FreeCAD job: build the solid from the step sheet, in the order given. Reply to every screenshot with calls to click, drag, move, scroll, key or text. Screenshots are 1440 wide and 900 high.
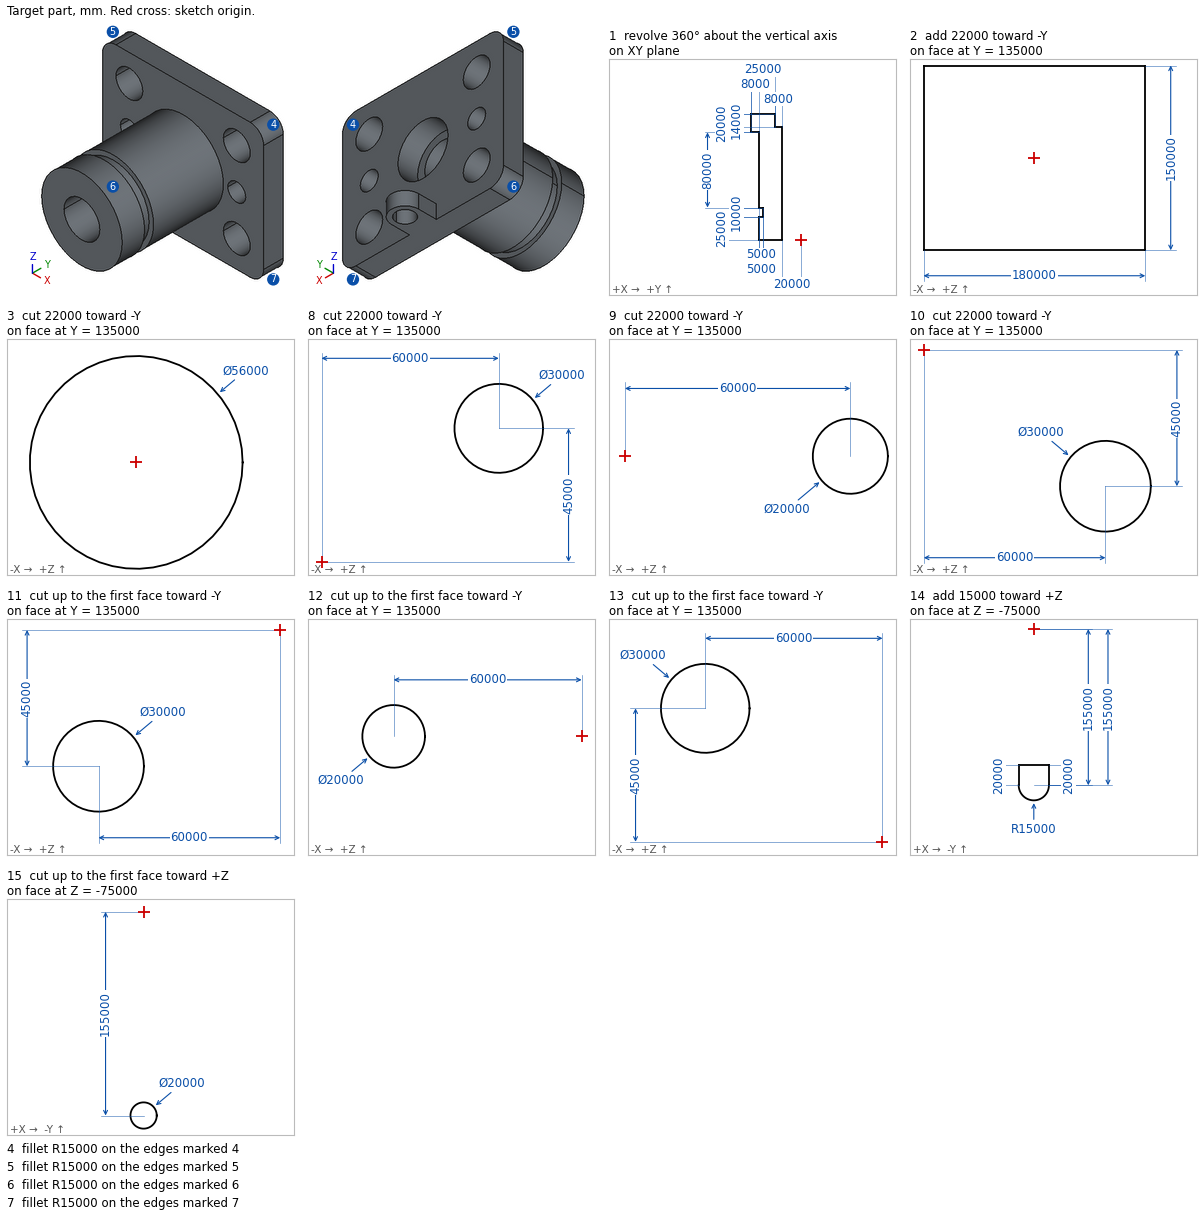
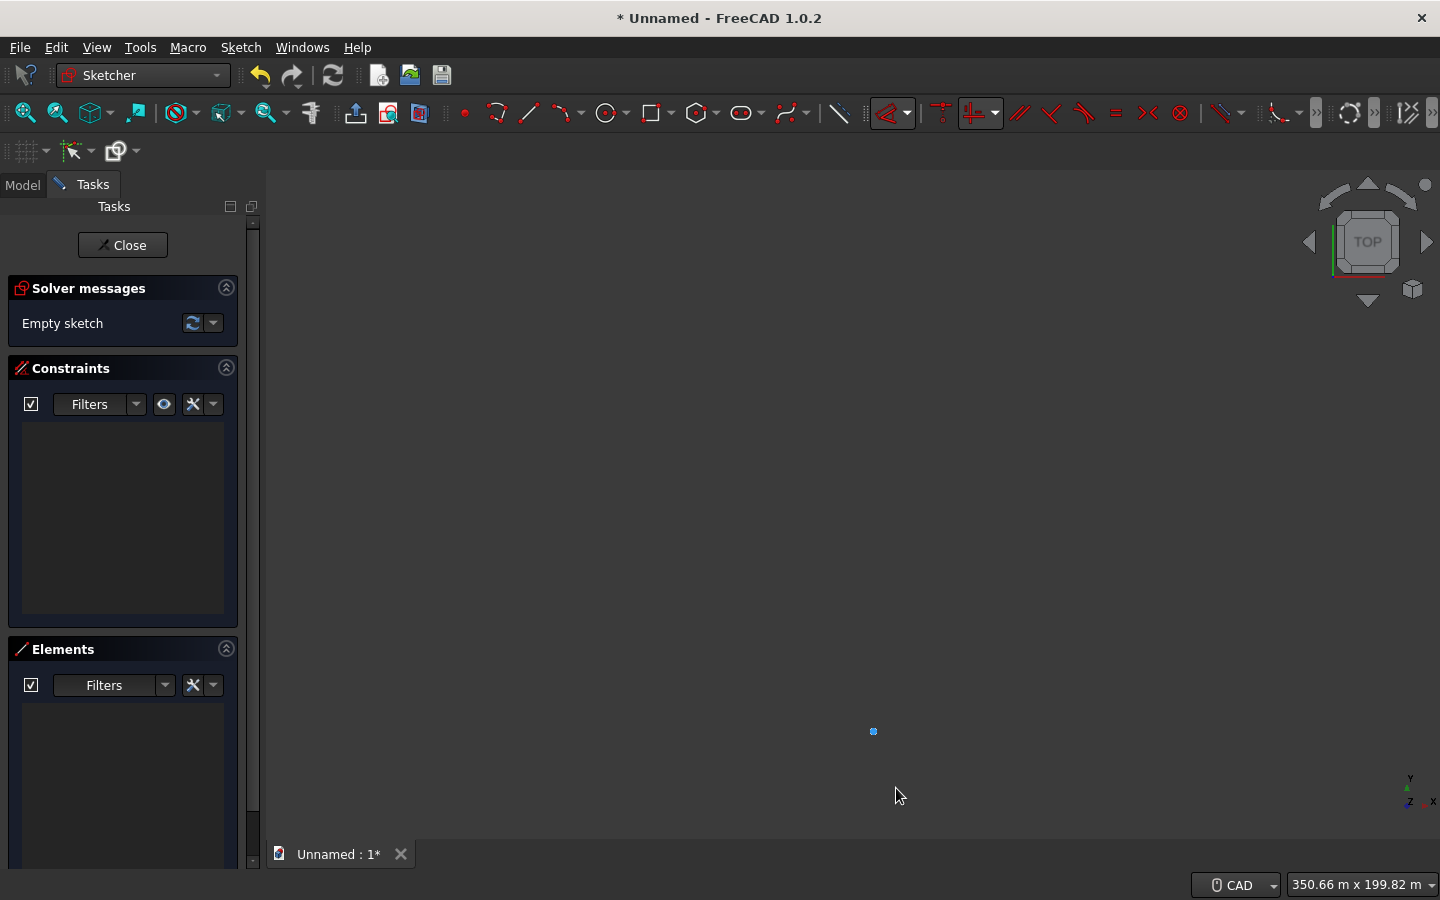
click(498, 114)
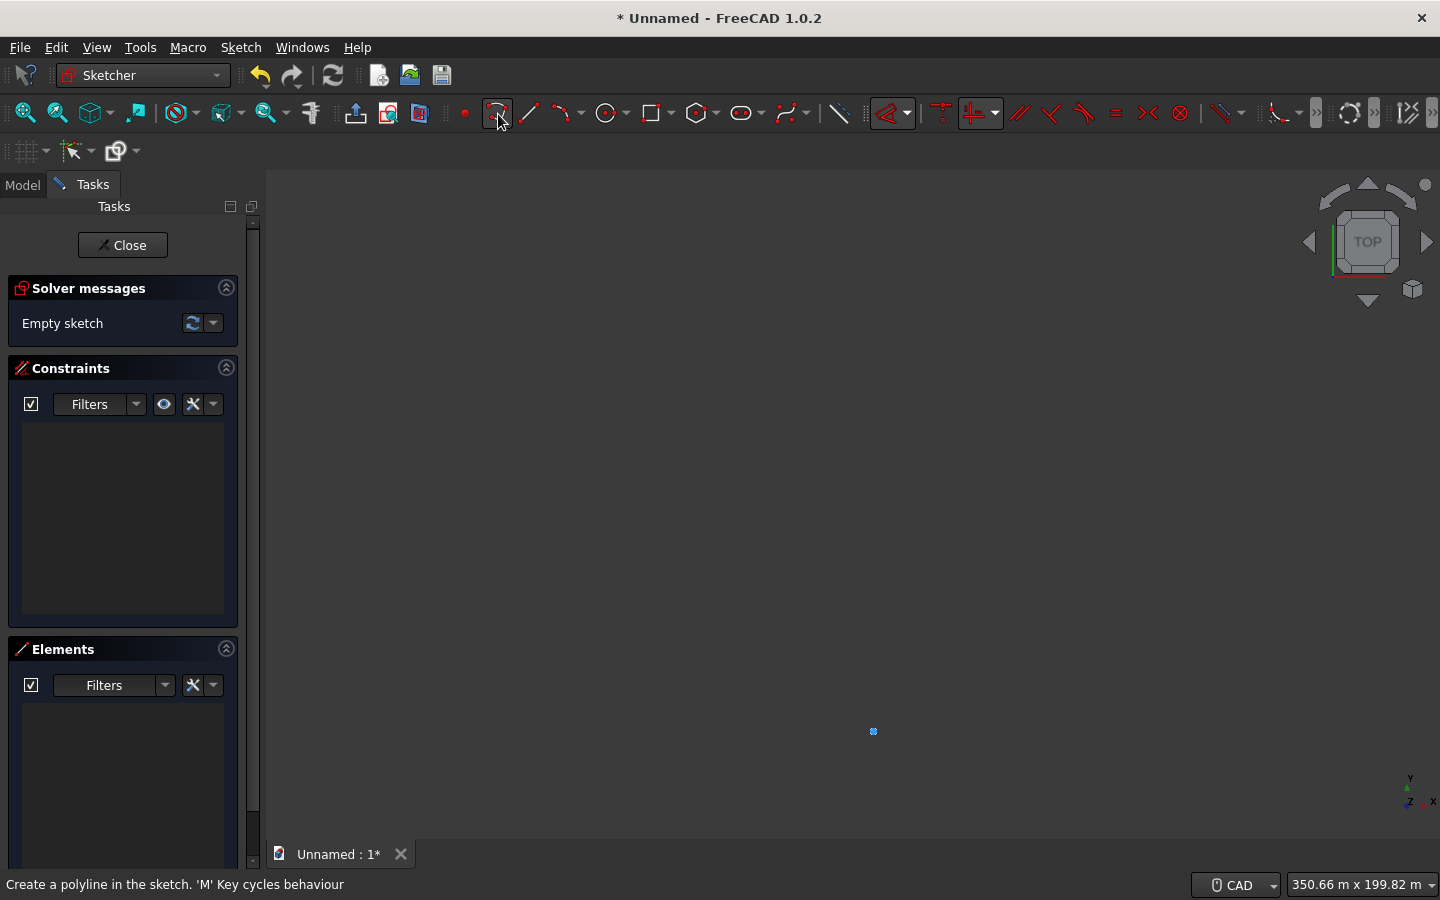
click(807, 732)
click(807, 326)
click(780, 326)
click(780, 280)
click(696, 280)
click(696, 346)
click(723, 346)
click(723, 614)
click(740, 614)
click(740, 648)
click(723, 648)
click(723, 723)
click(807, 733)
key(Escape)
key(Escape)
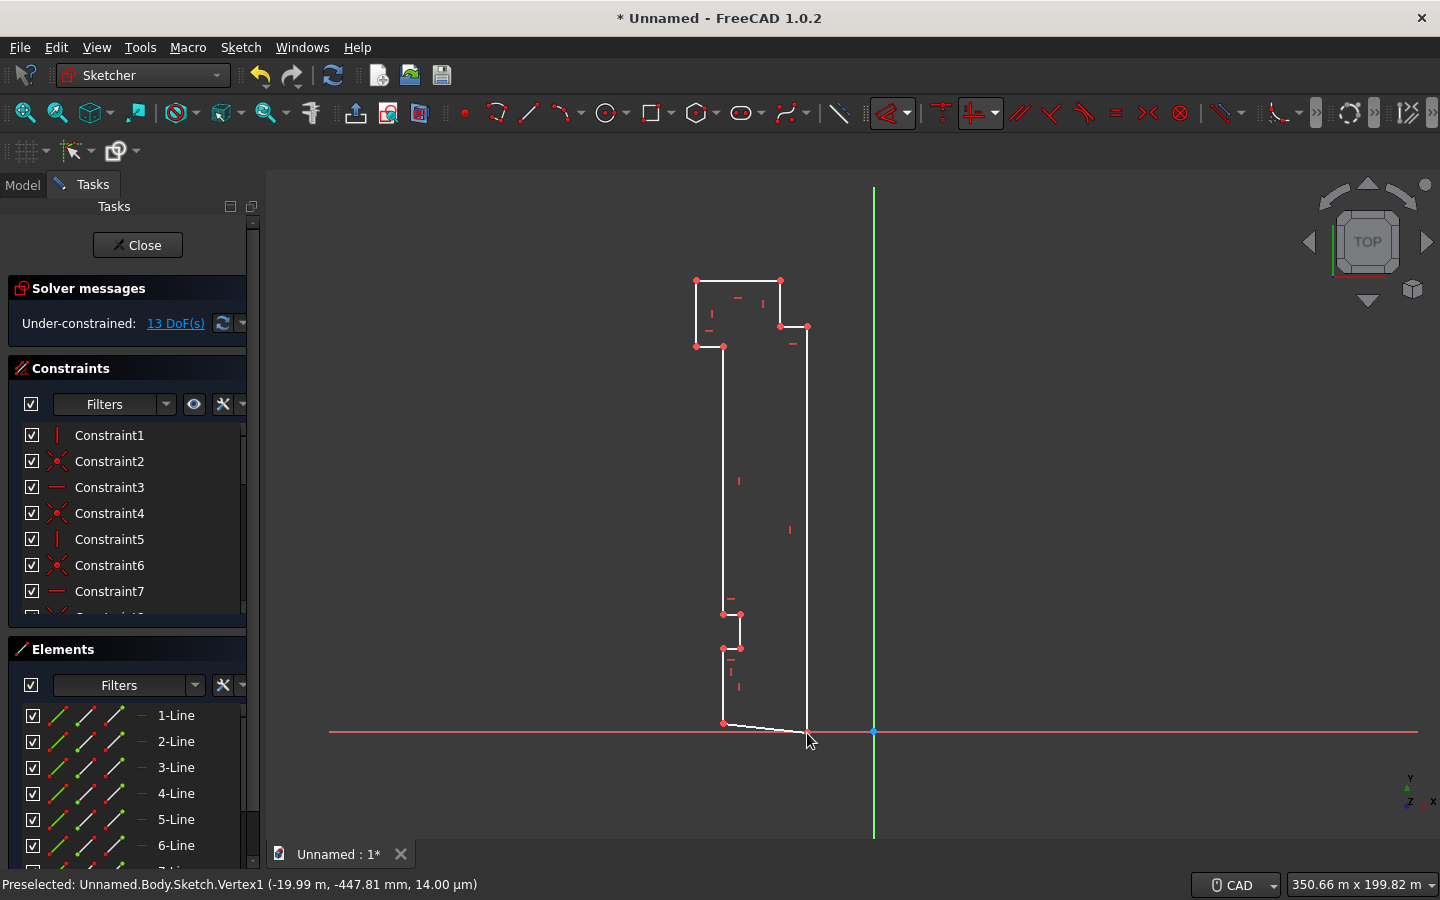
click(782, 730)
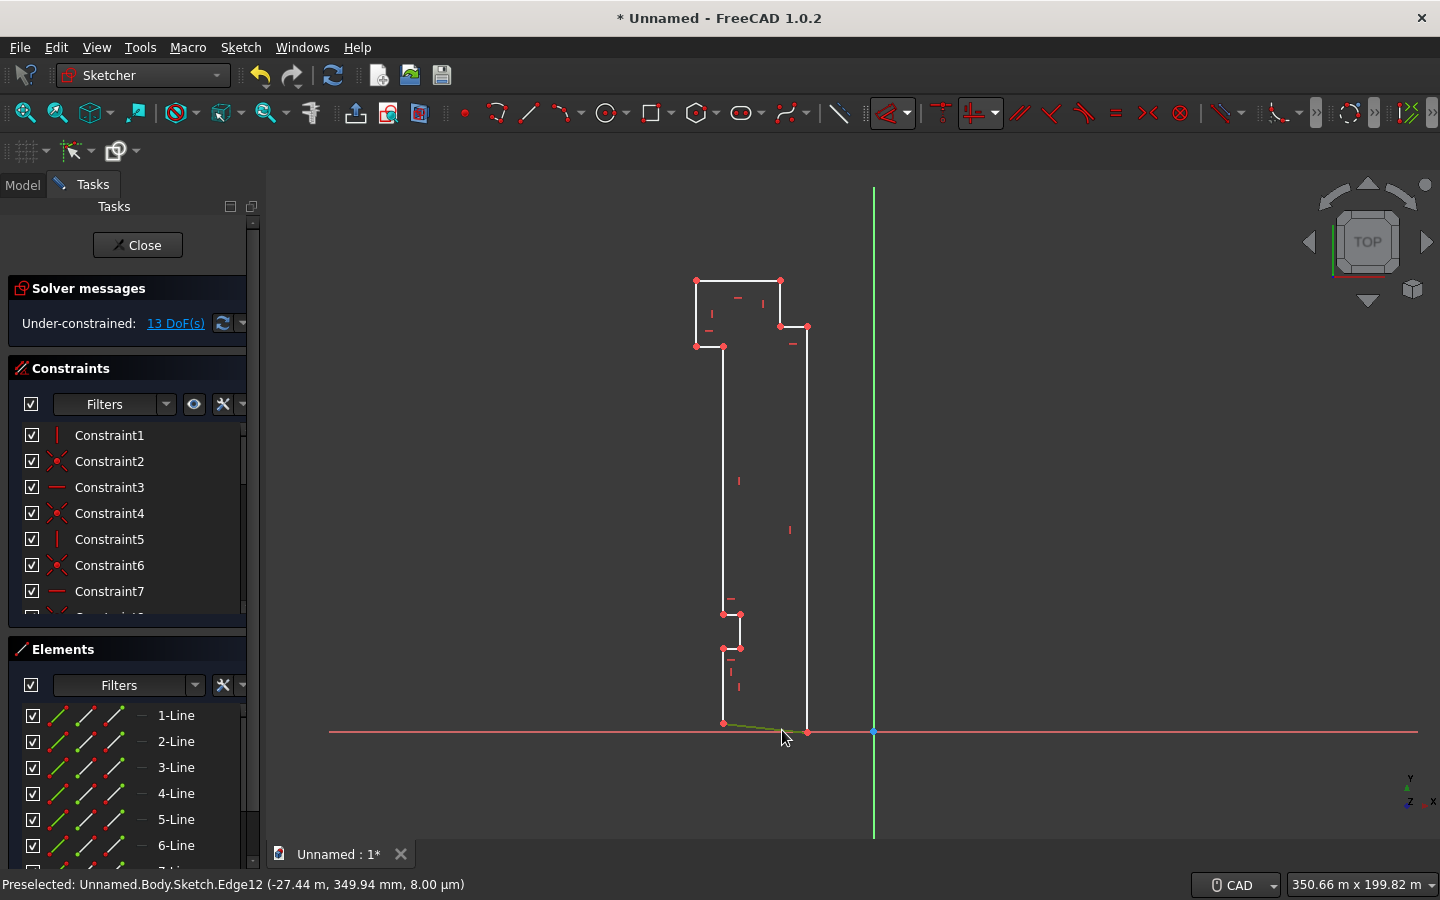
click(998, 114)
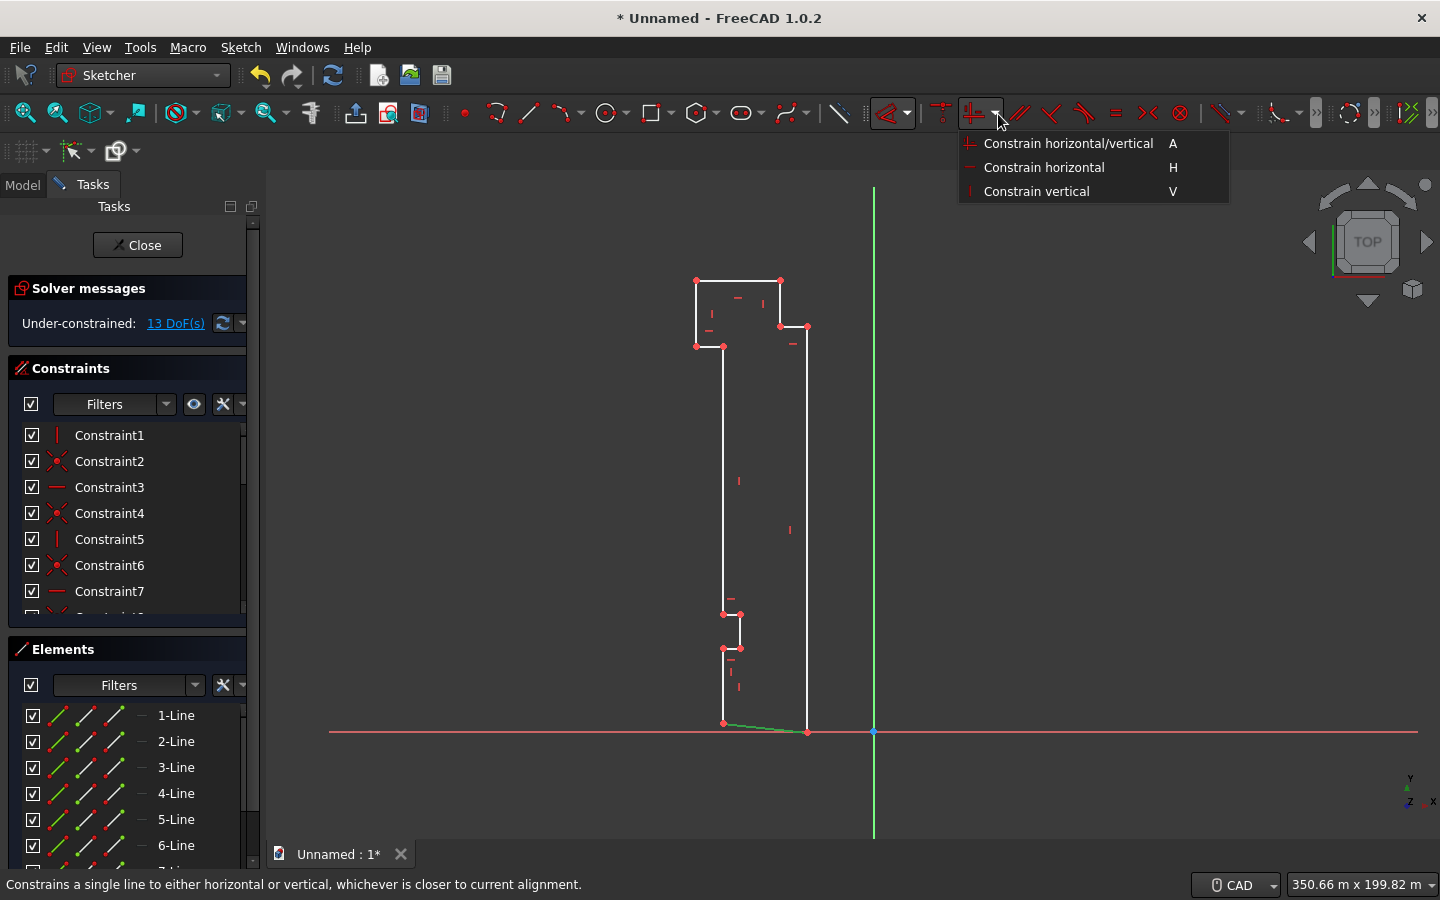
click(1094, 167)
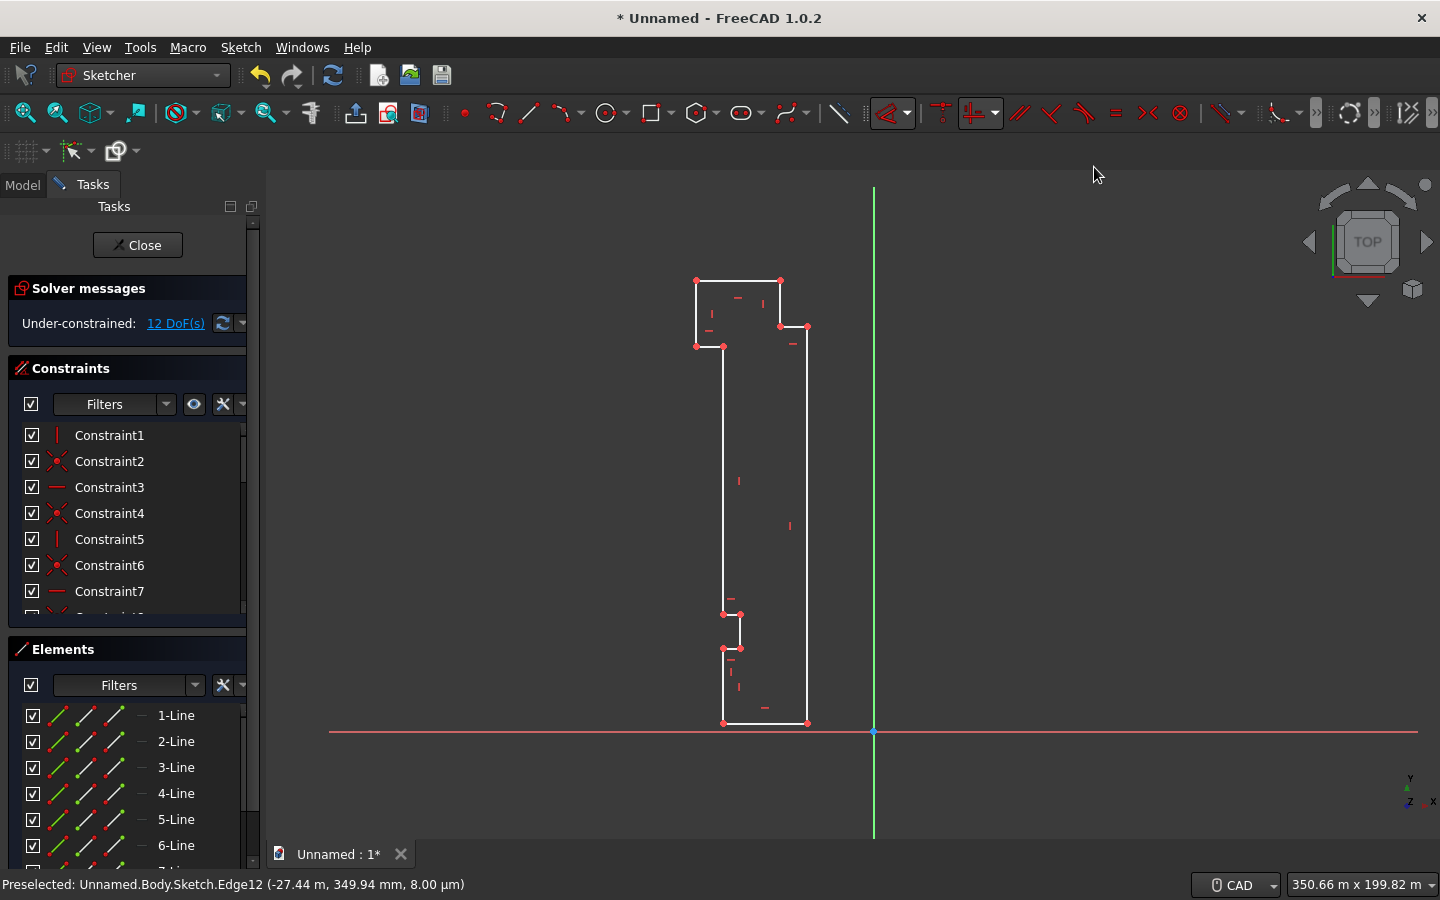
click(807, 724)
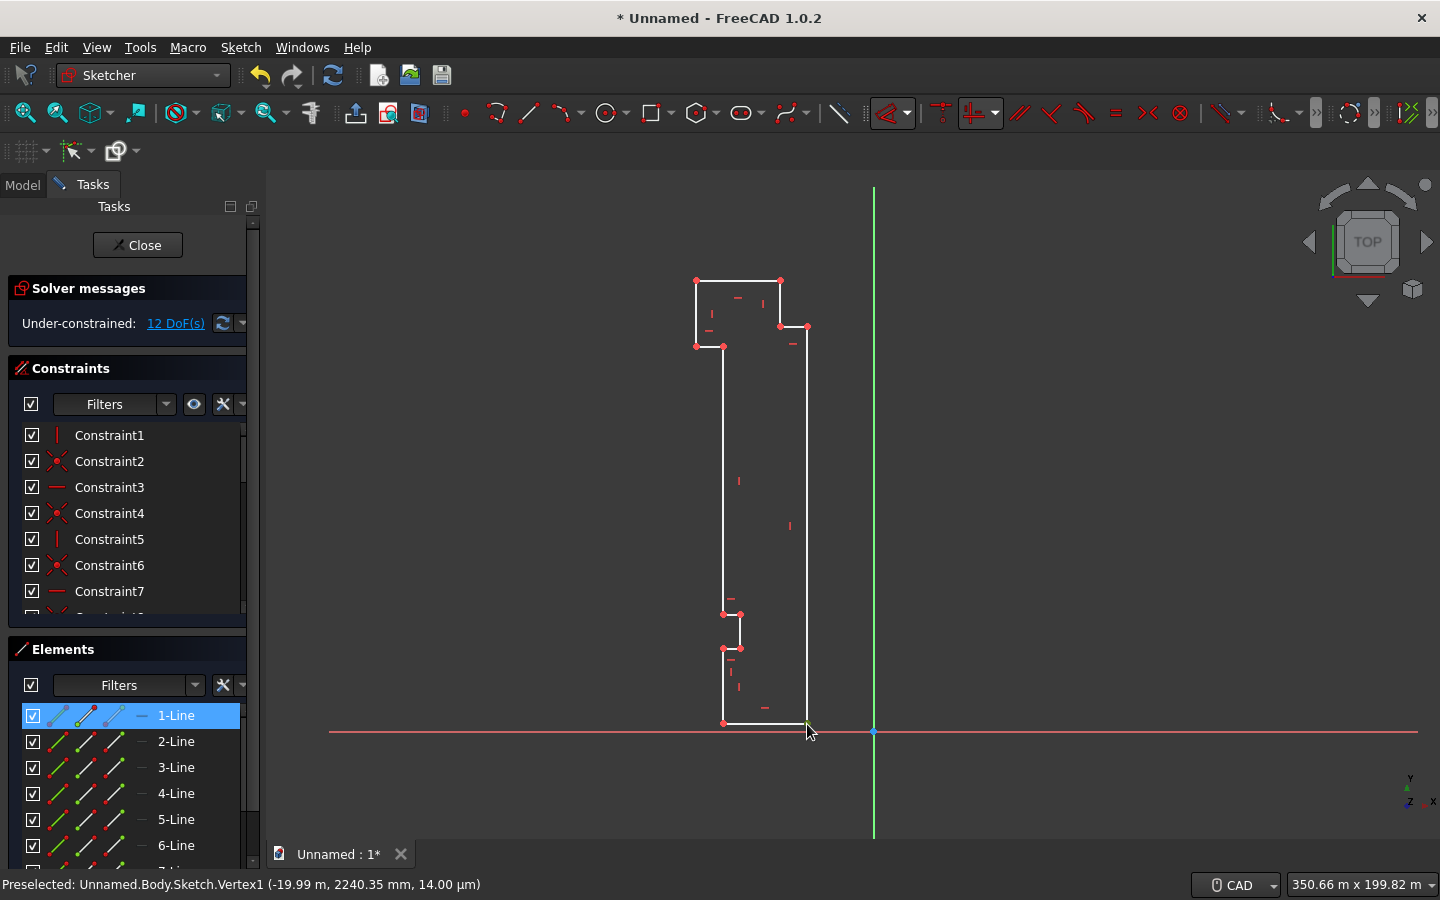
click(364, 732)